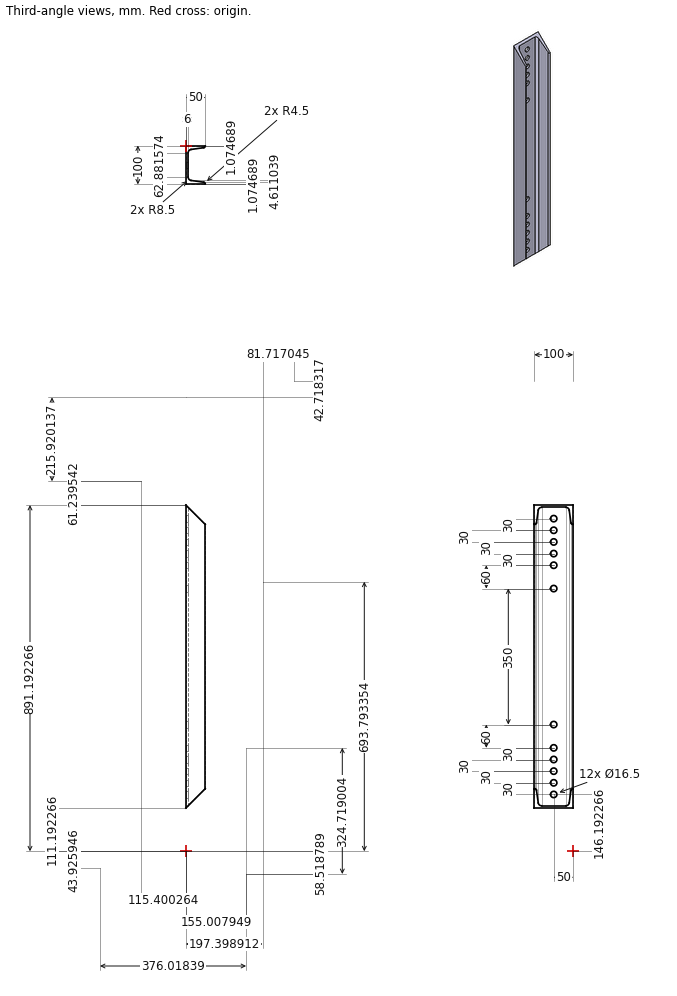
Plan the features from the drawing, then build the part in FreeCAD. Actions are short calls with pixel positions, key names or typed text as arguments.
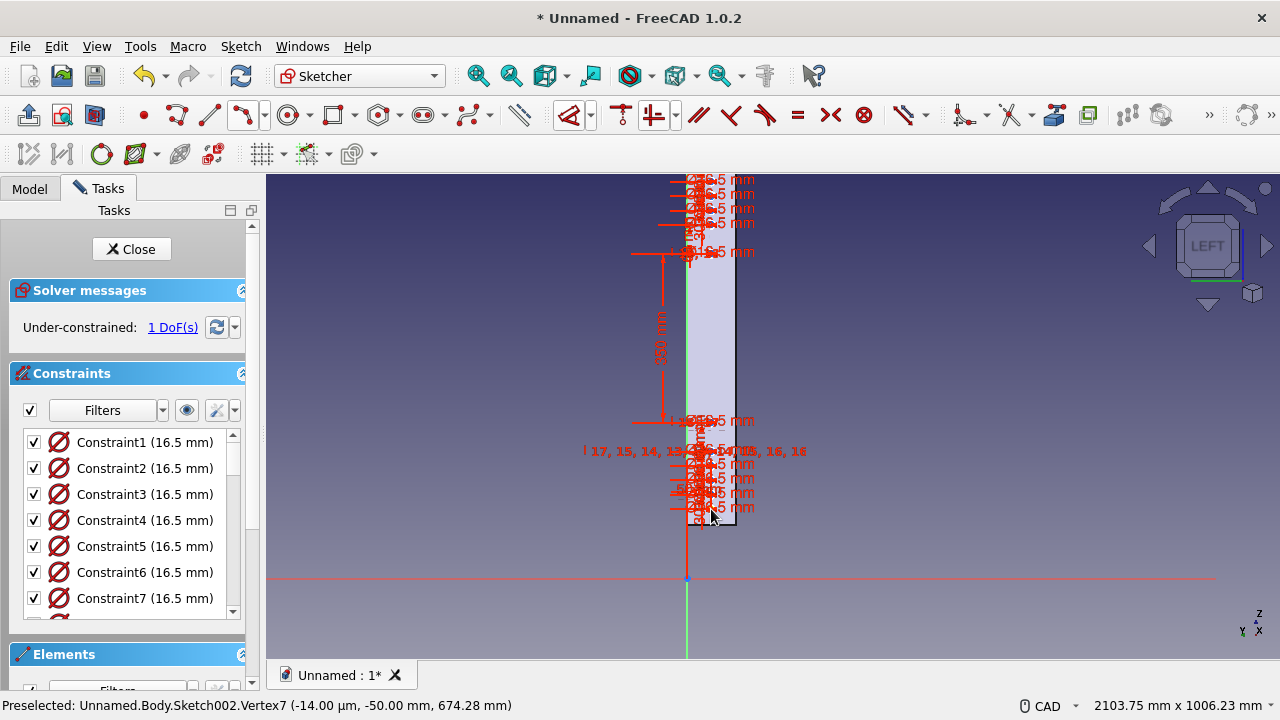
click(711, 509)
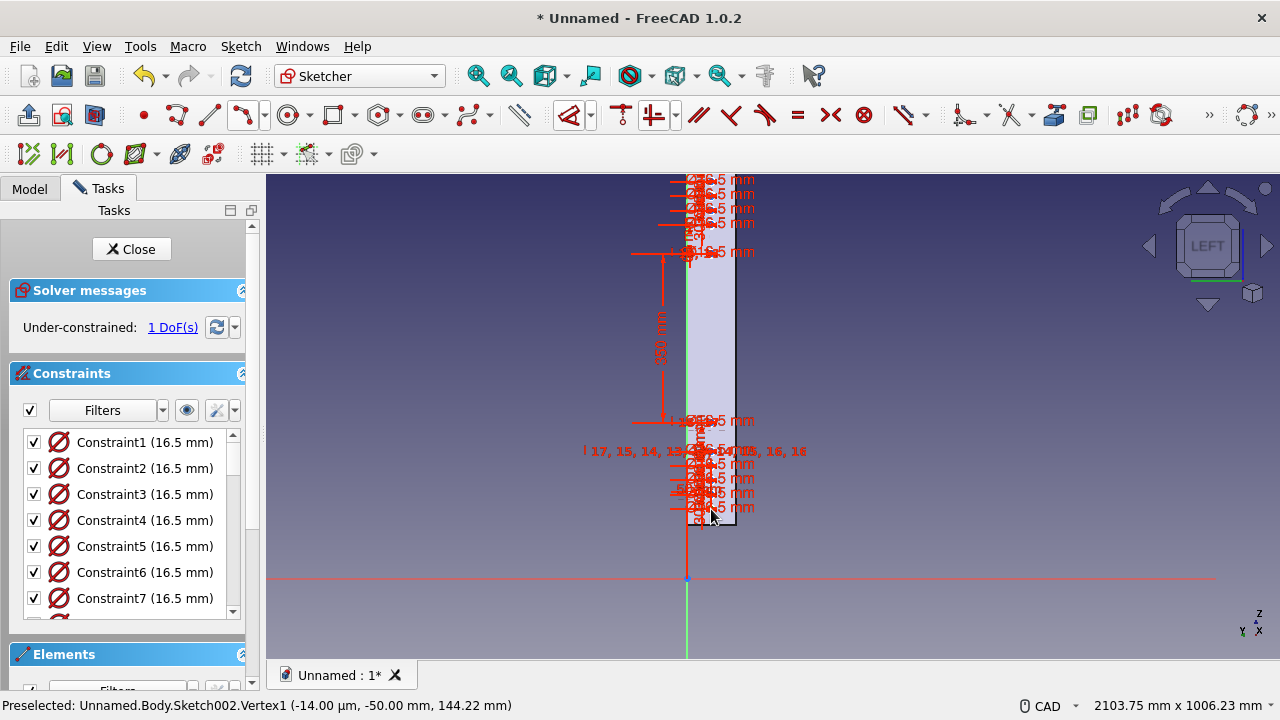
click(590, 116)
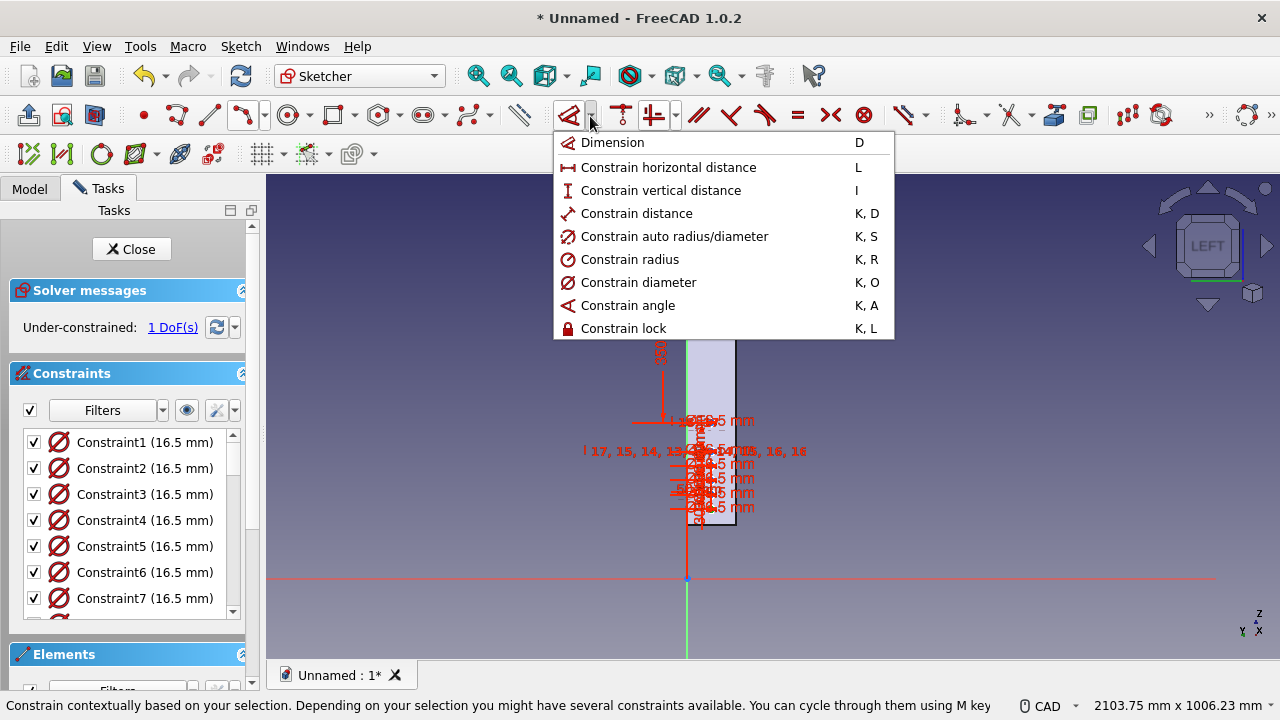
click(724, 190)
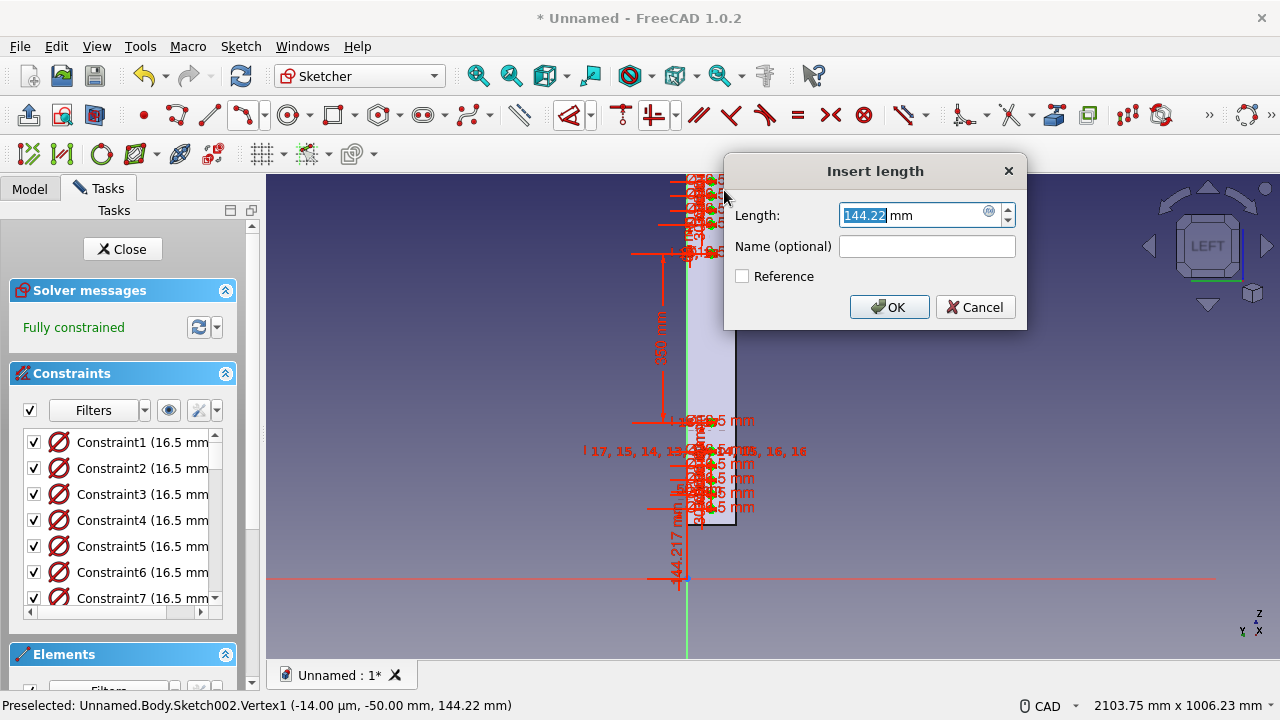
text(146.192266)
key(Return)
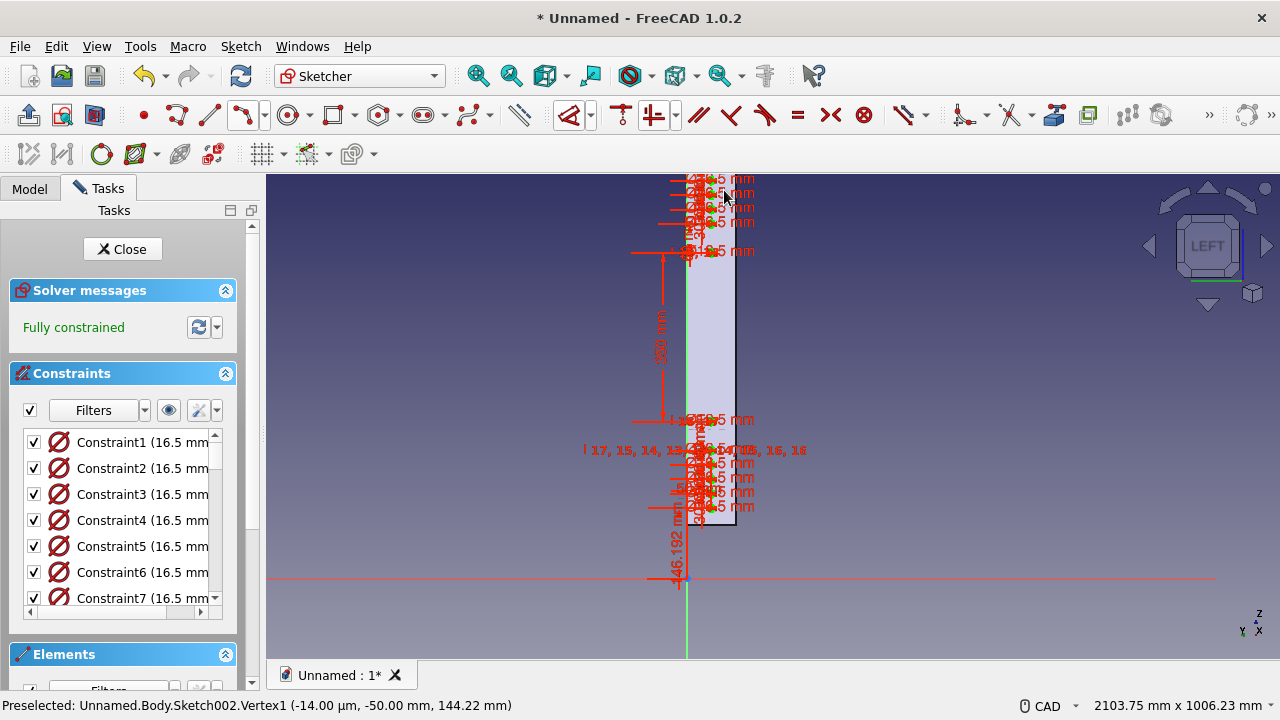
click(123, 249)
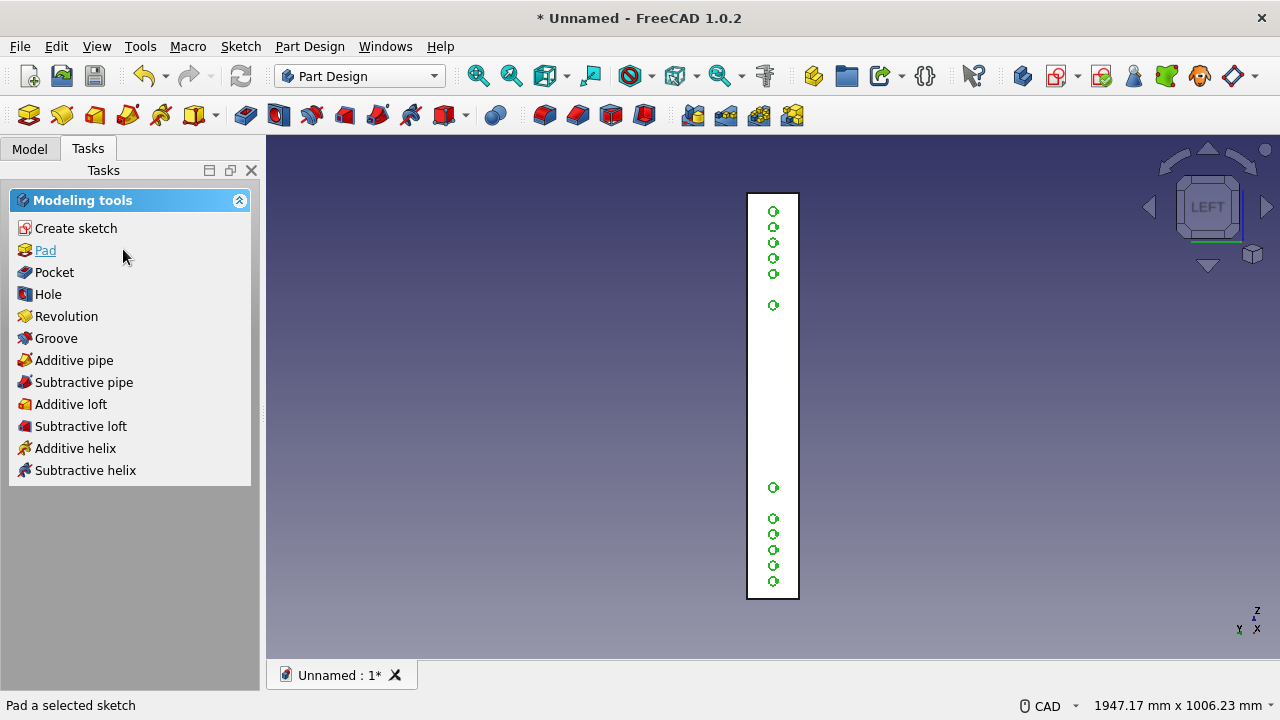
click(246, 116)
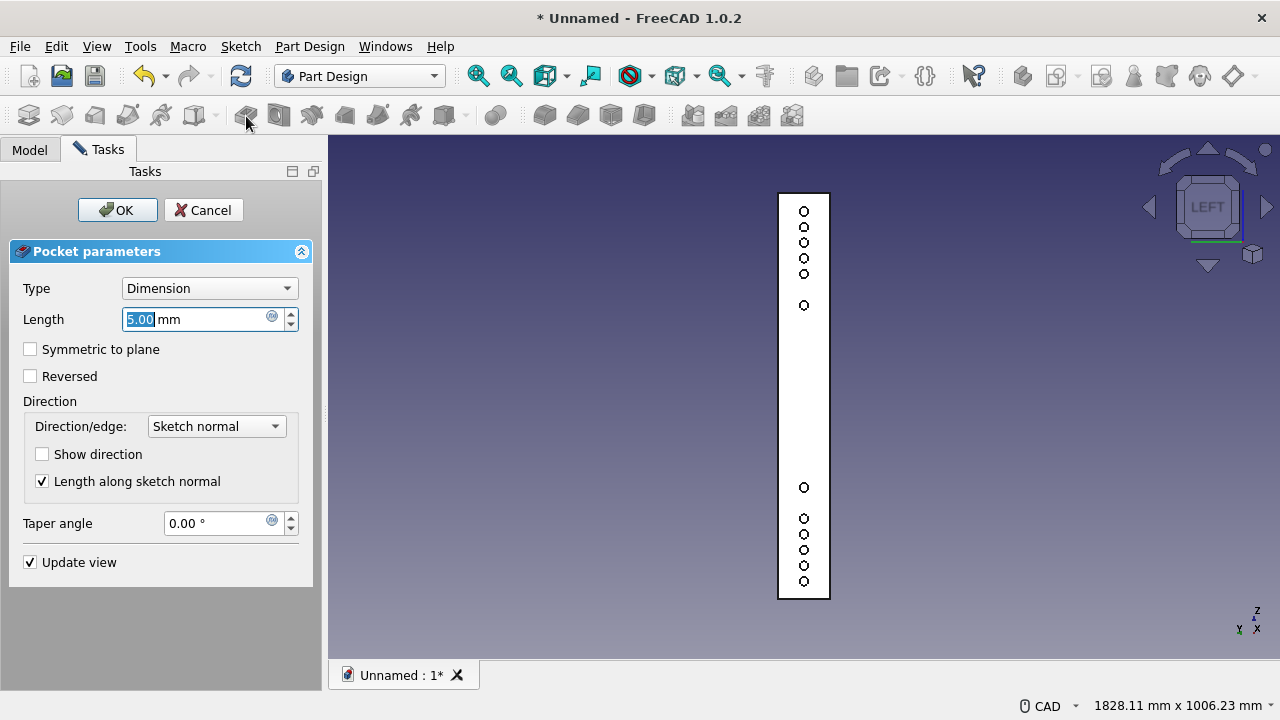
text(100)
key(Tab)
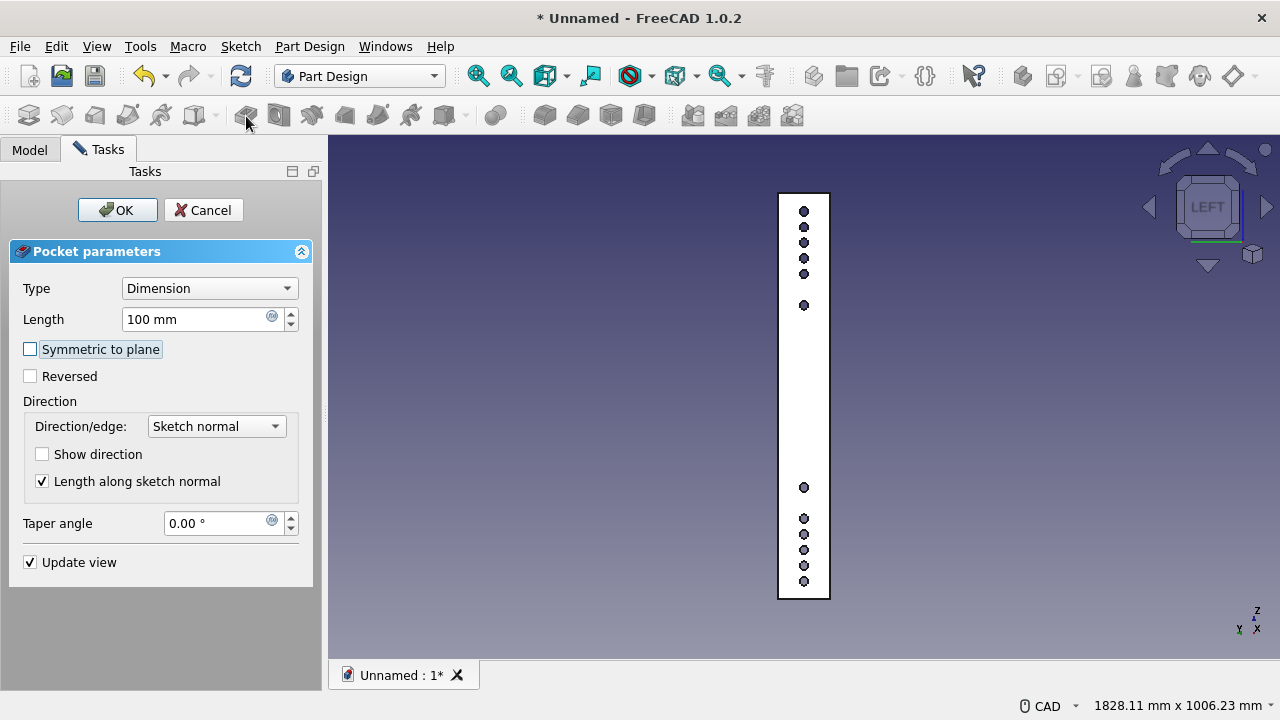
click(118, 210)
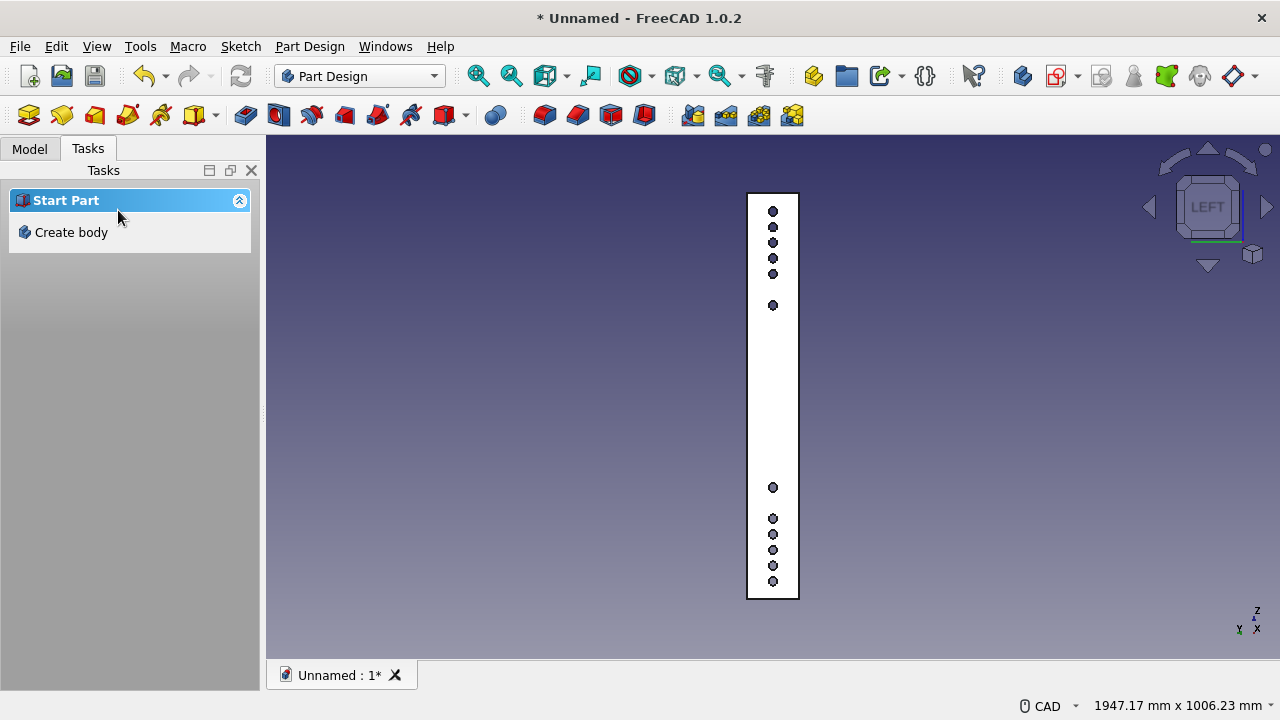
key(0)